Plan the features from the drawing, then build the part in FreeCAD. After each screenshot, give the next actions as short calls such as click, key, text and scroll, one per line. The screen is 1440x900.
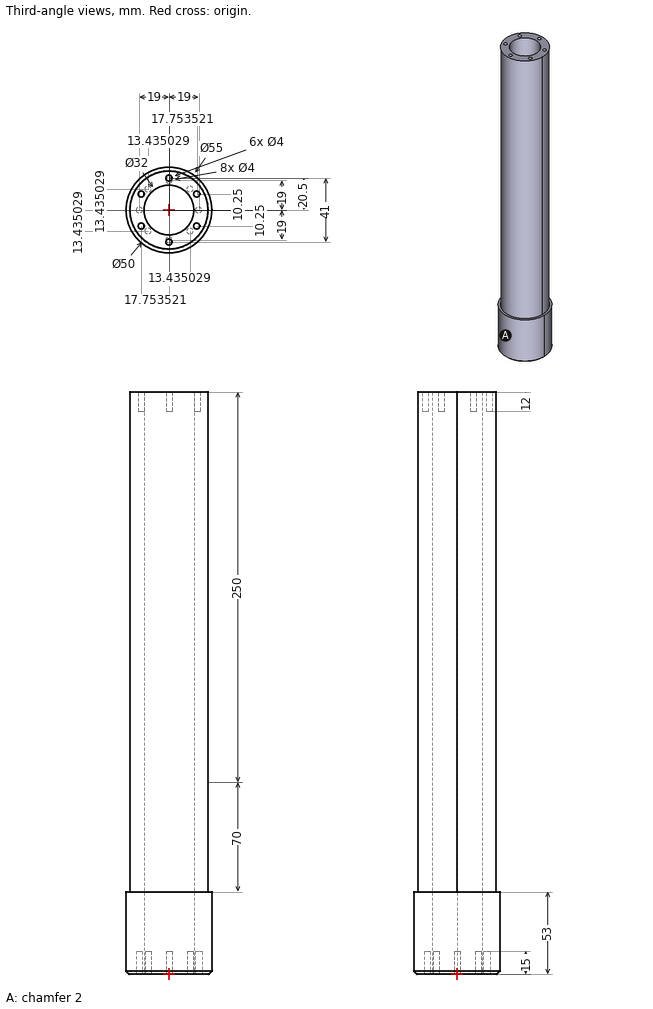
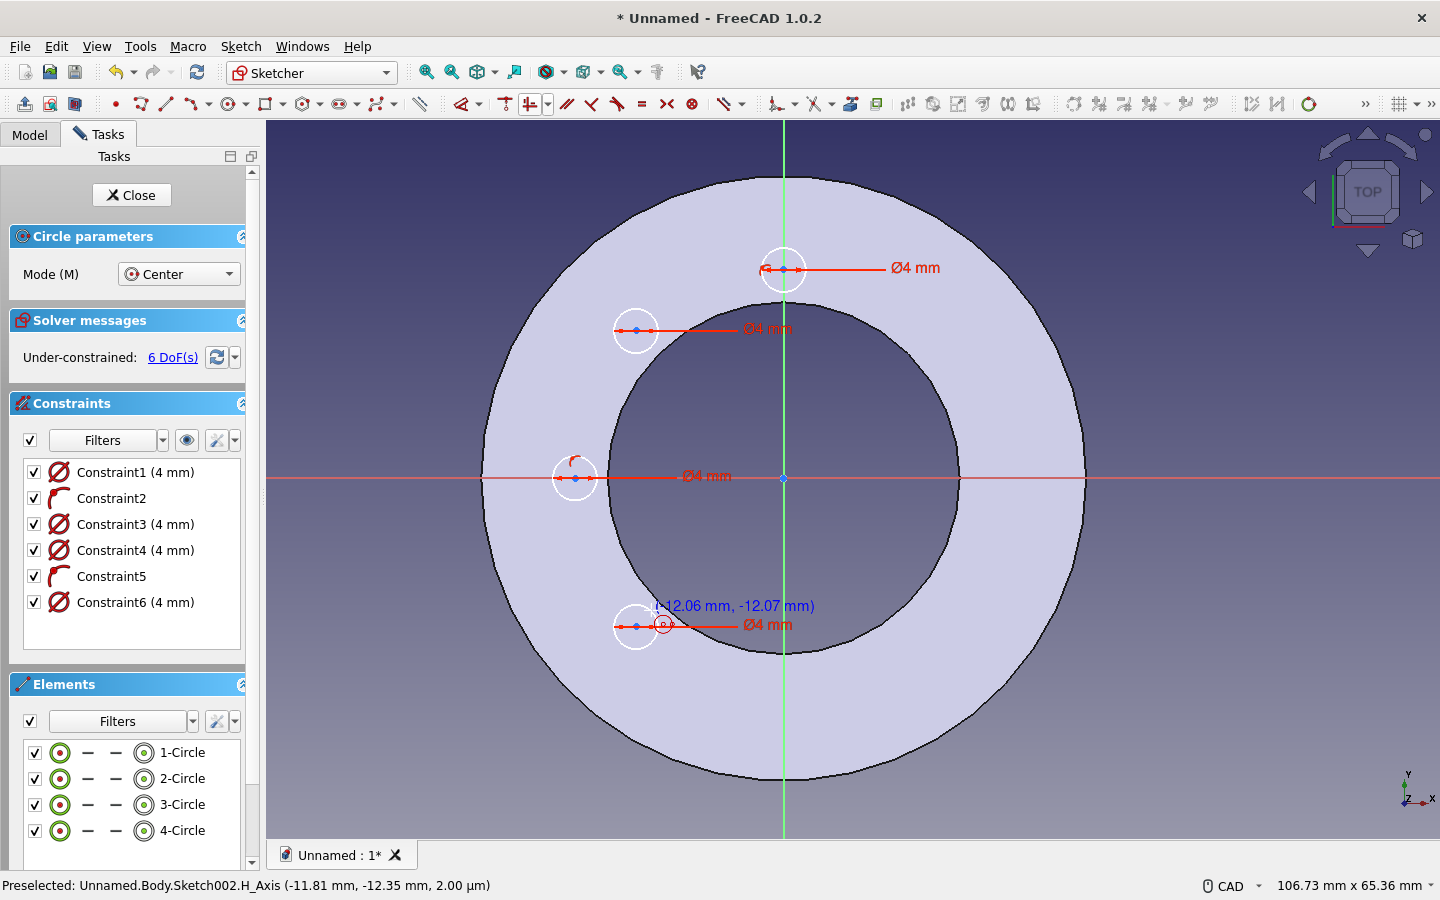
click(784, 687)
move(799, 672)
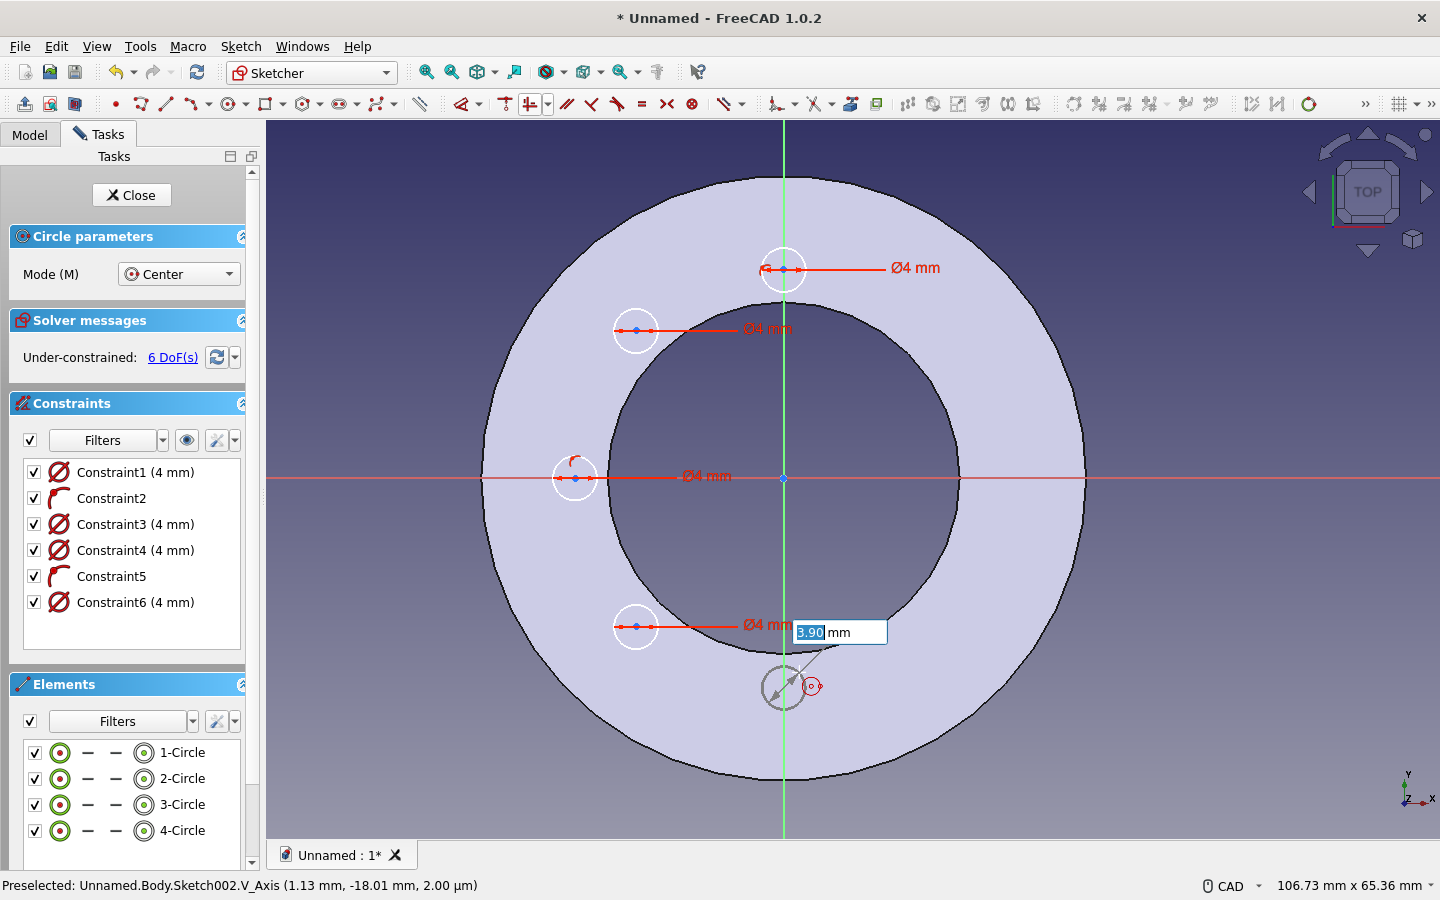
text(4)
key(Return)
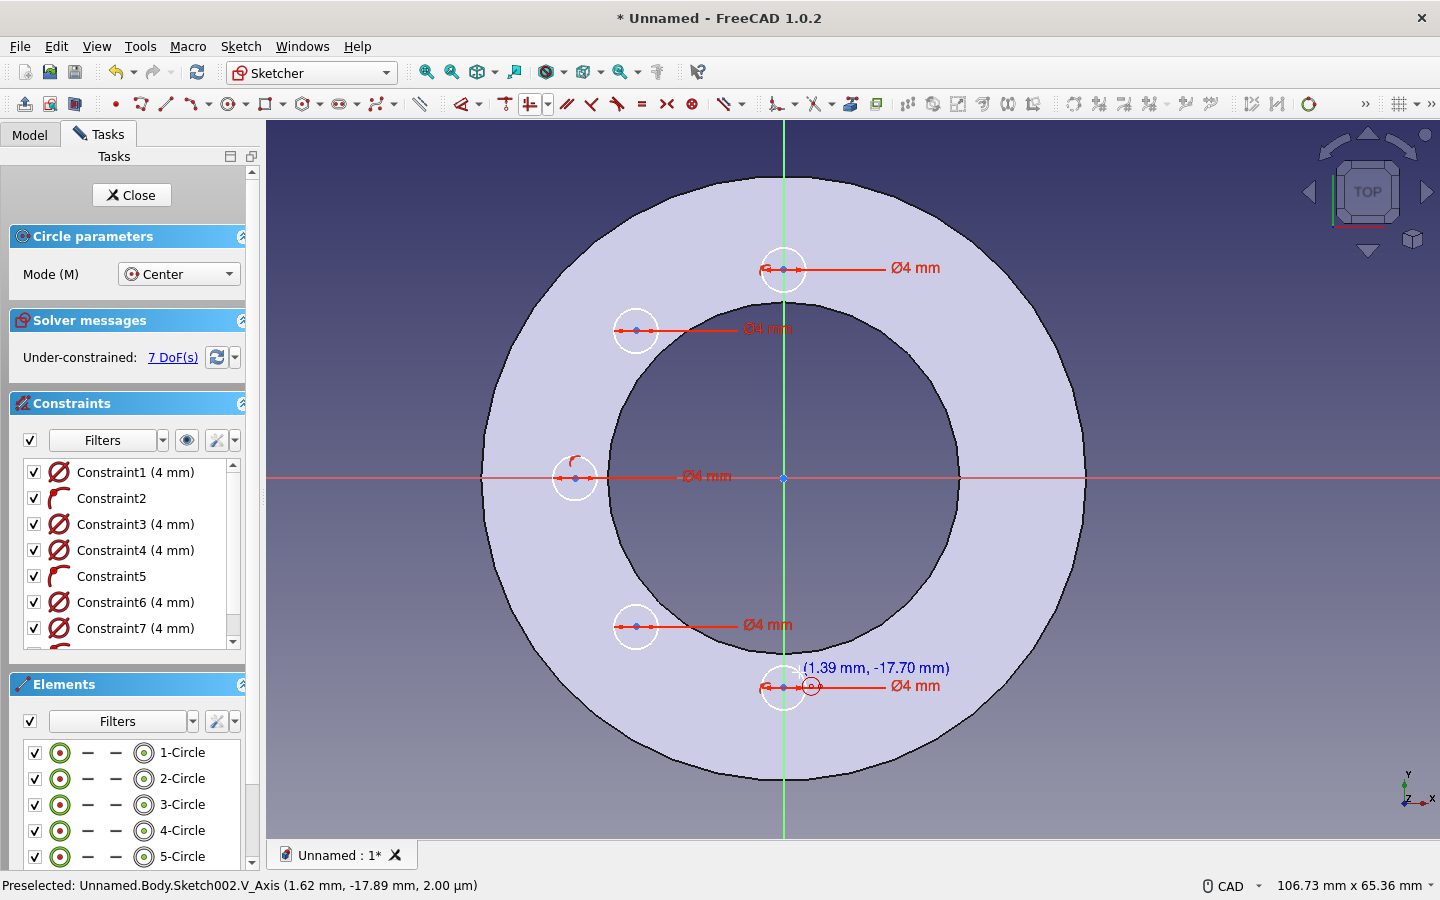
click(931, 626)
move(947, 610)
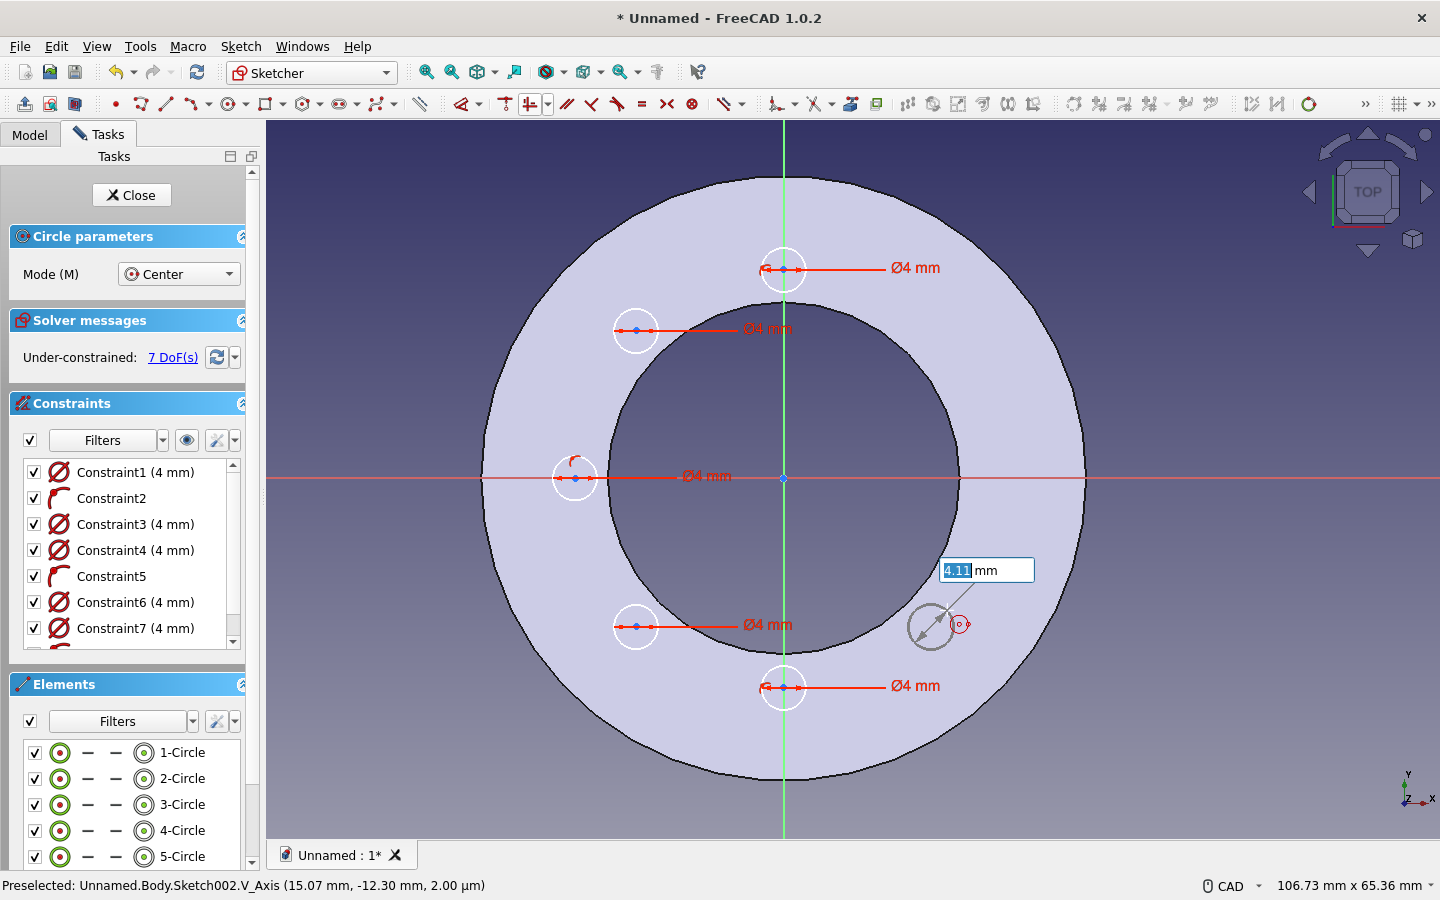
text(4)
key(Return)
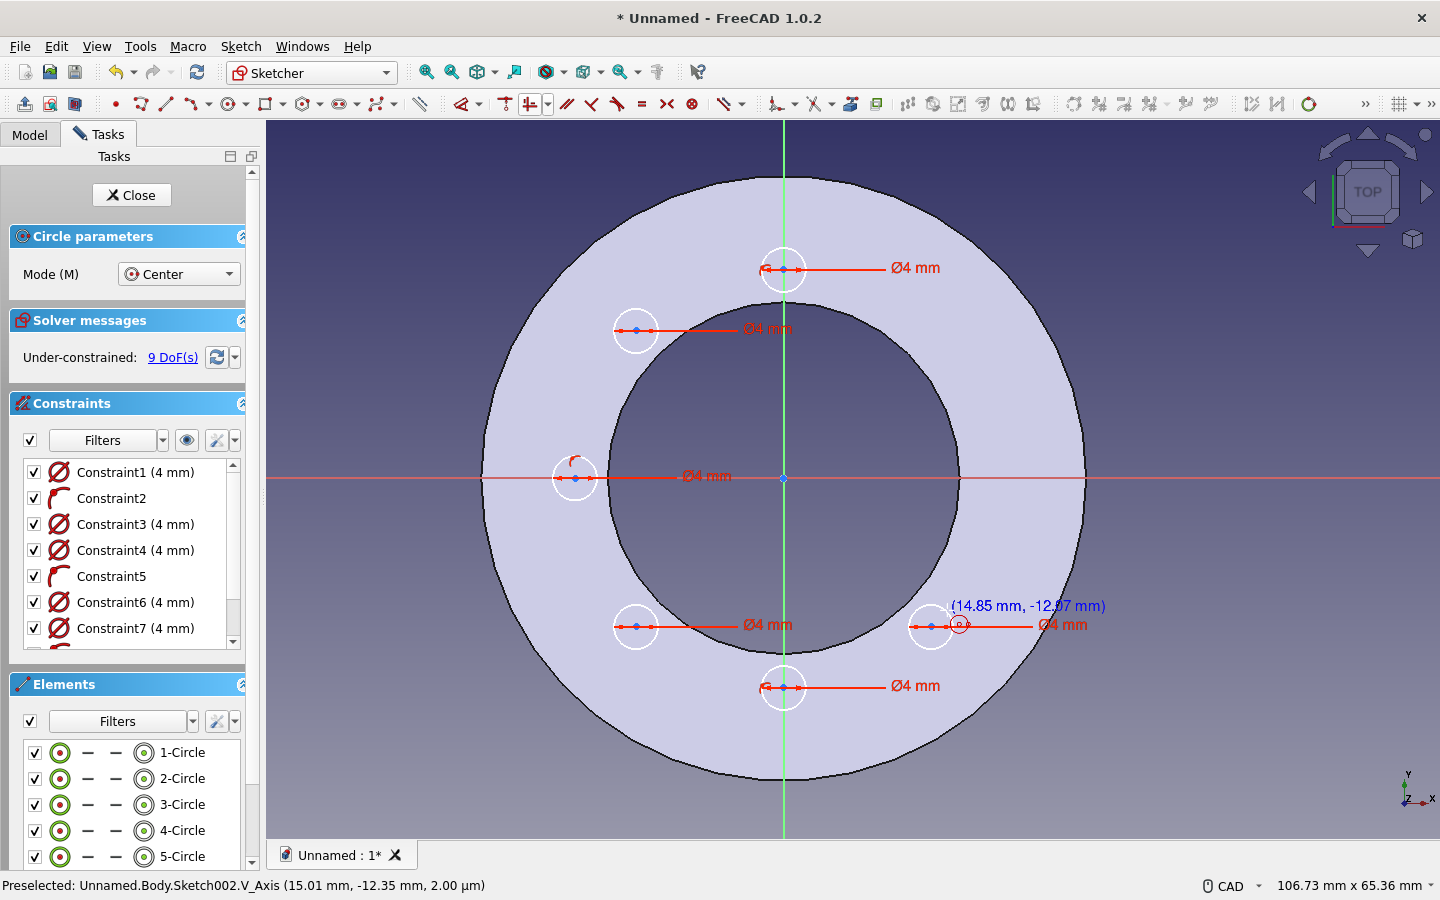
click(993, 478)
move(1008, 463)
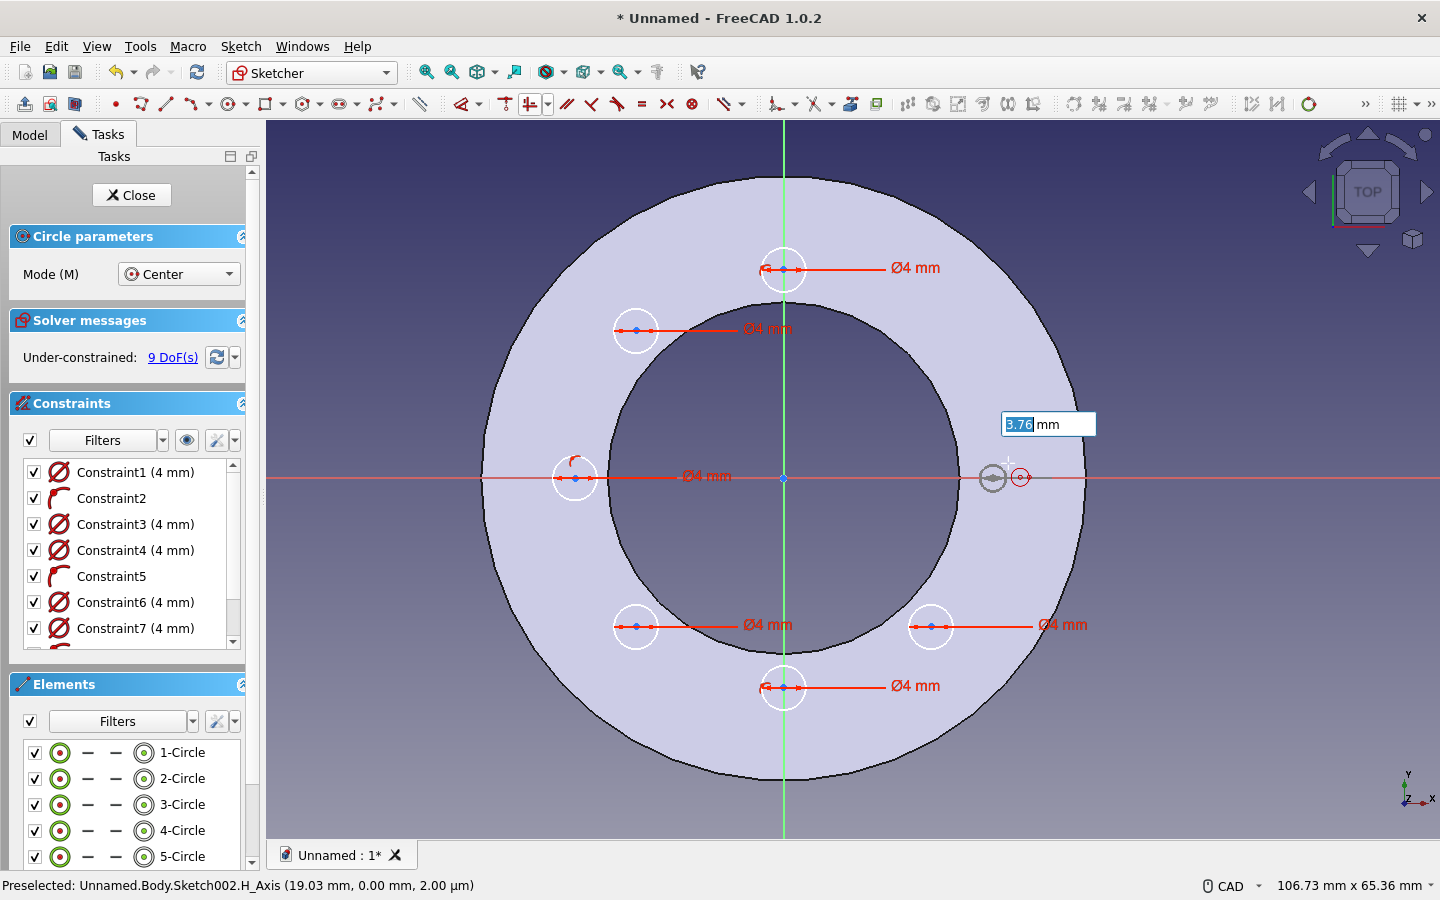
text(4)
key(Return)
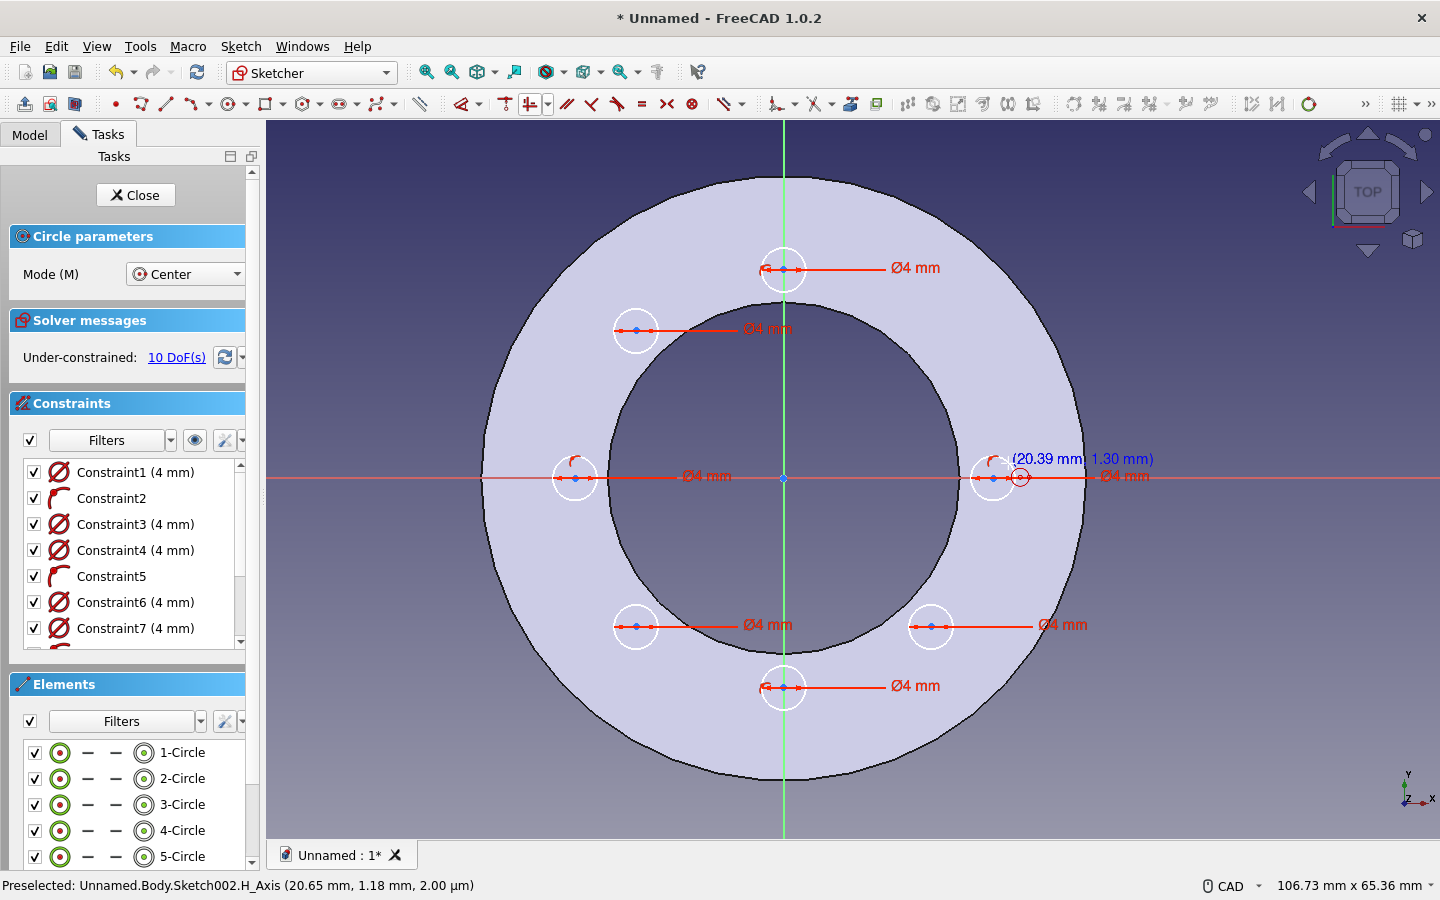
click(931, 330)
move(947, 315)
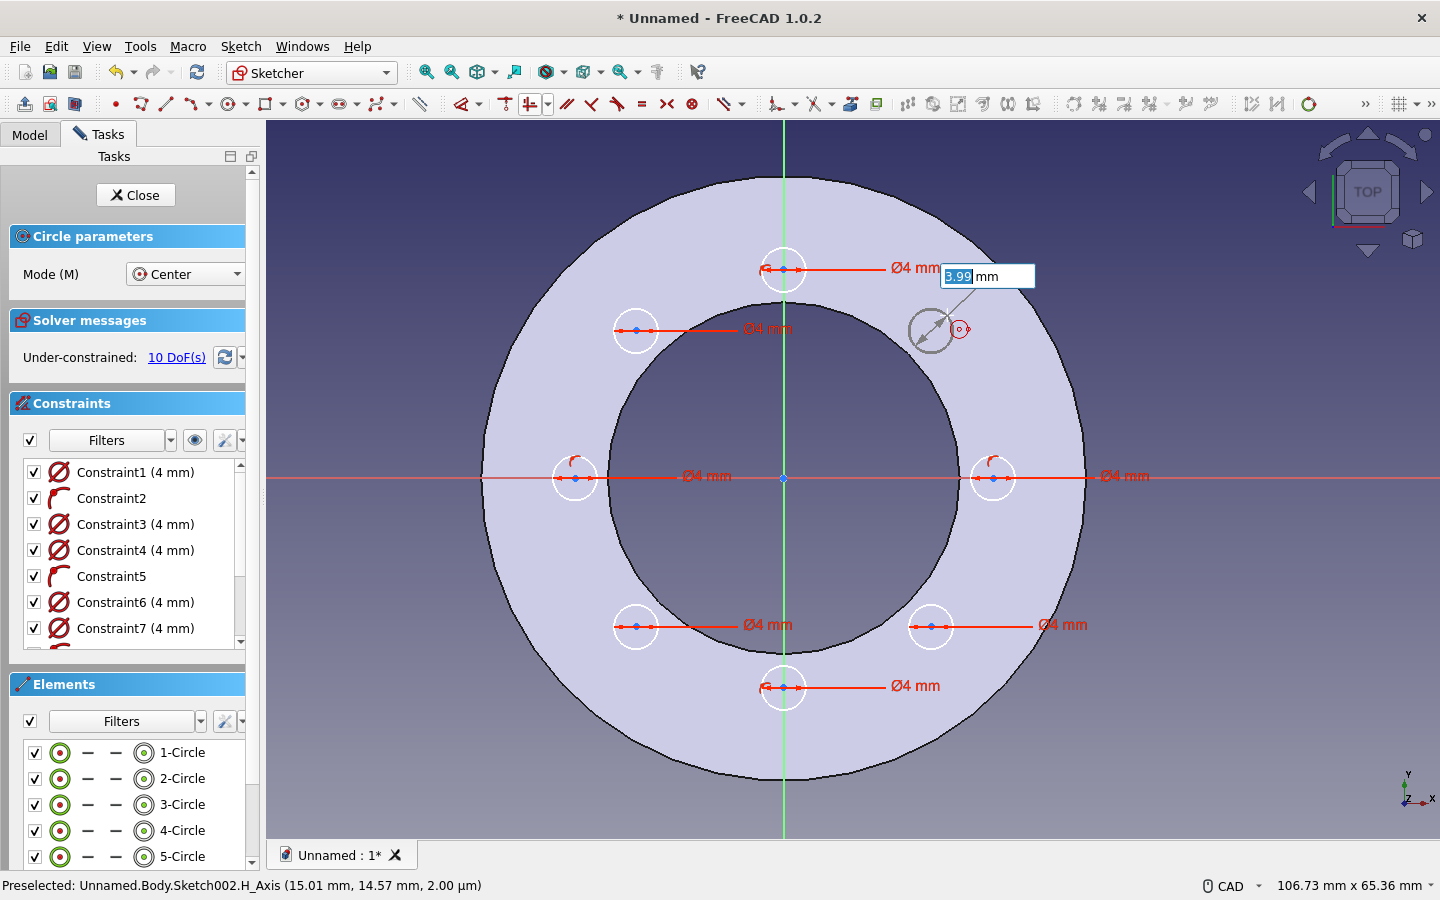
text(4)
key(Return)
key(Escape)